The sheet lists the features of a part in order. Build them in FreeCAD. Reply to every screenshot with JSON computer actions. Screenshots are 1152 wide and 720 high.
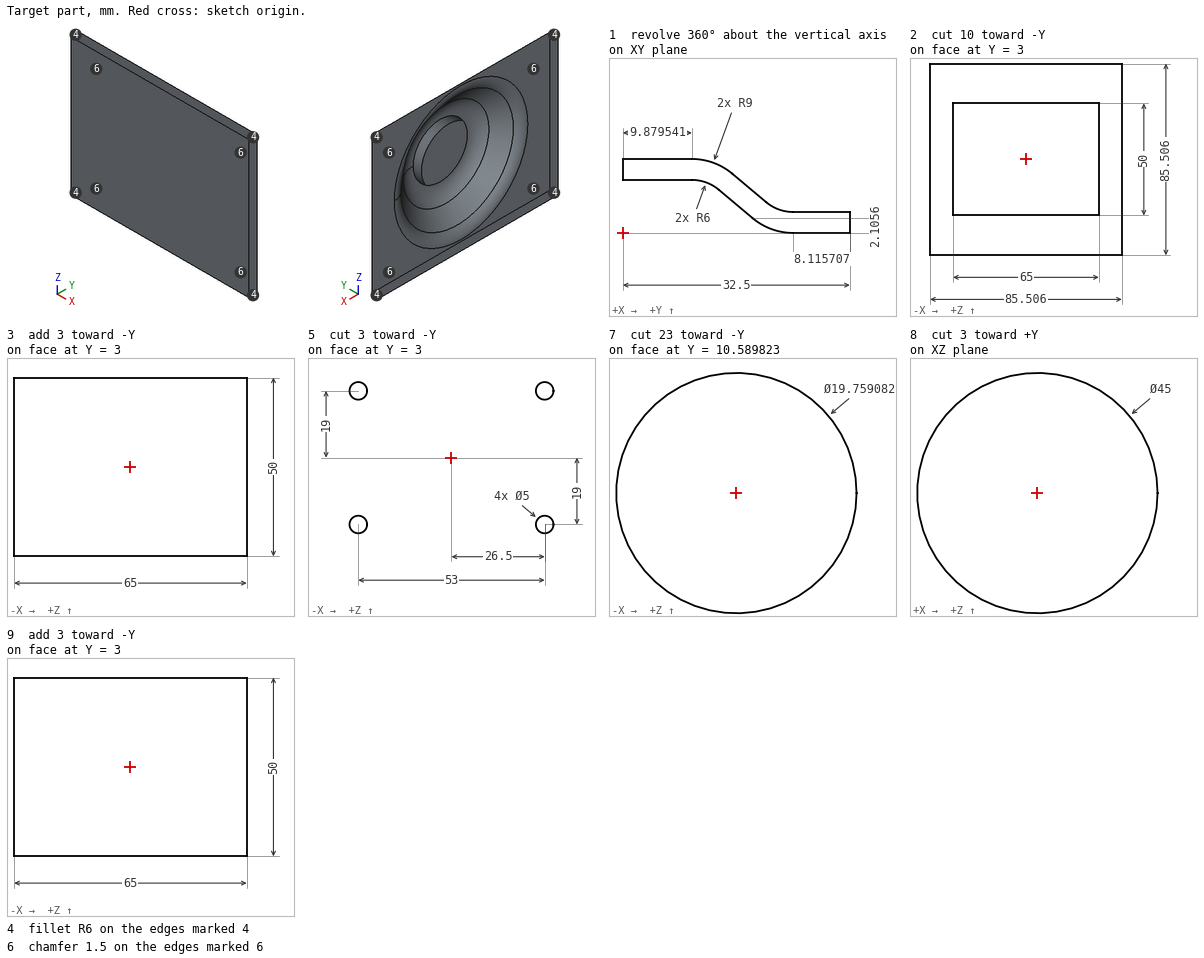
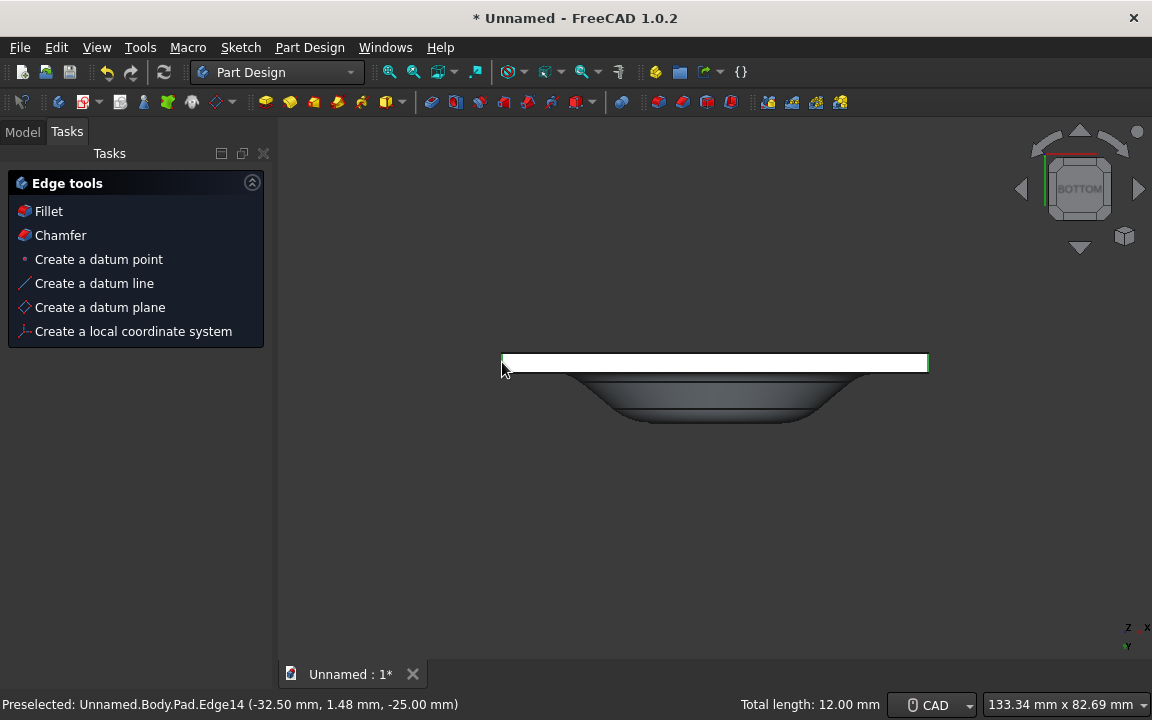
{"action": "left_click", "coordinate": [660, 102]}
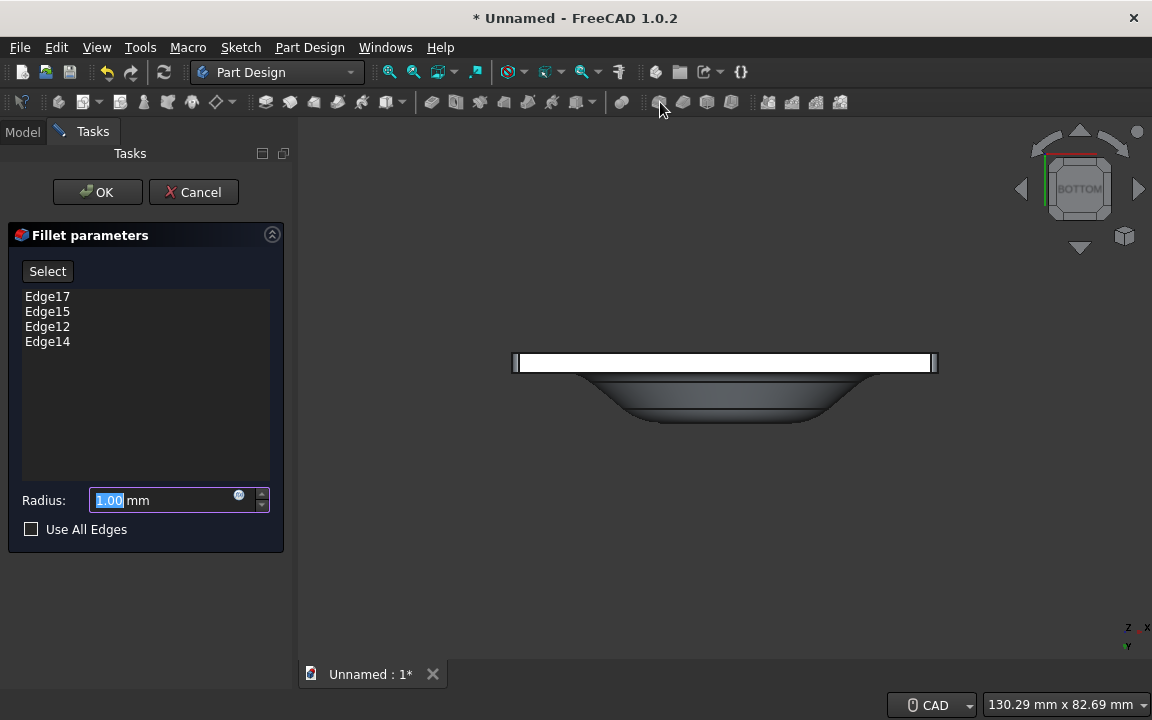
{"action": "type", "text": "6"}
{"action": "key", "text": "Tab"}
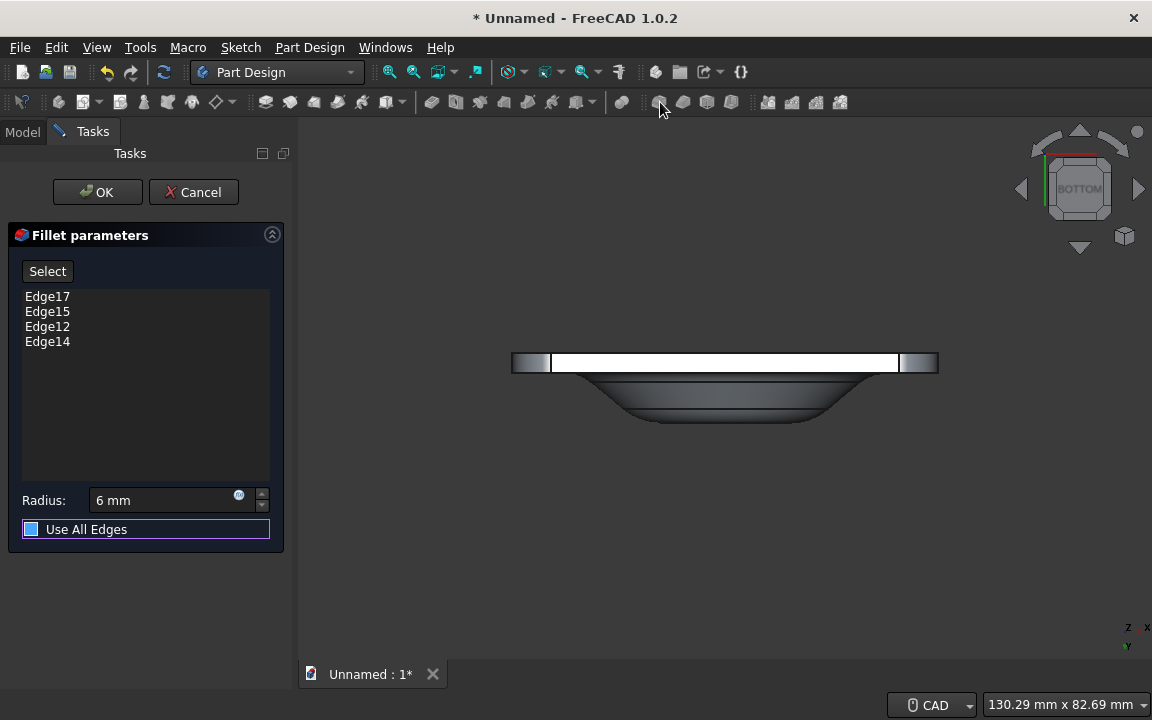
{"action": "left_click", "coordinate": [98, 192]}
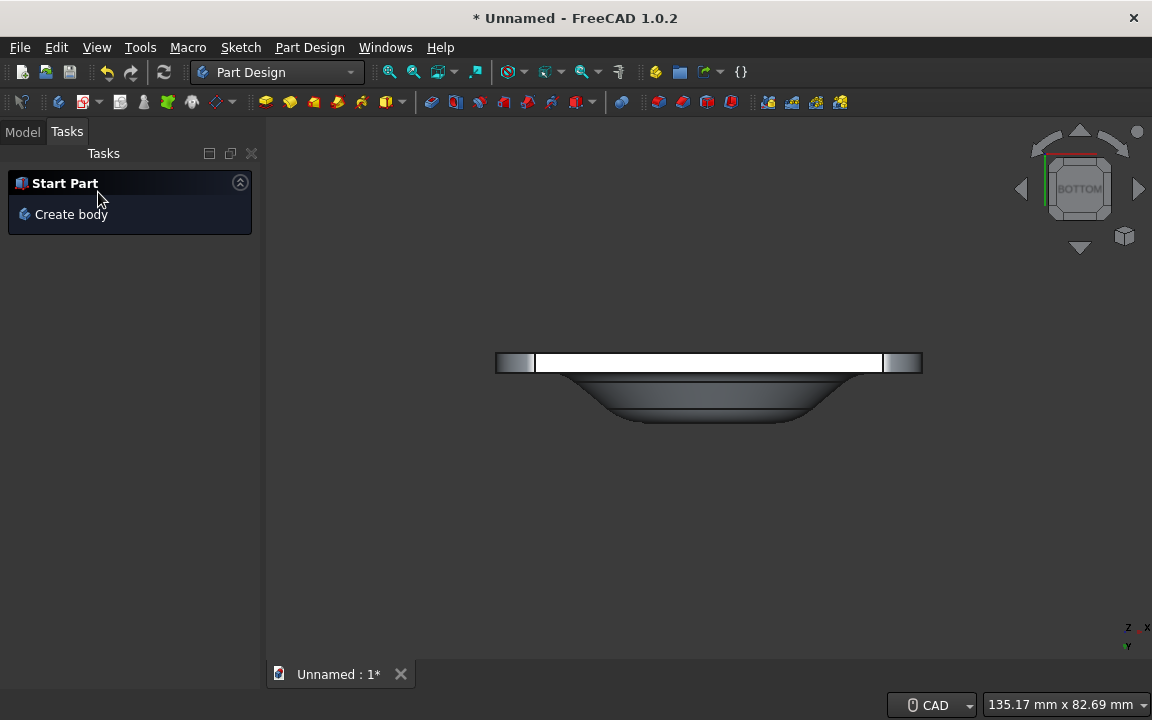
{"action": "key", "text": "4"}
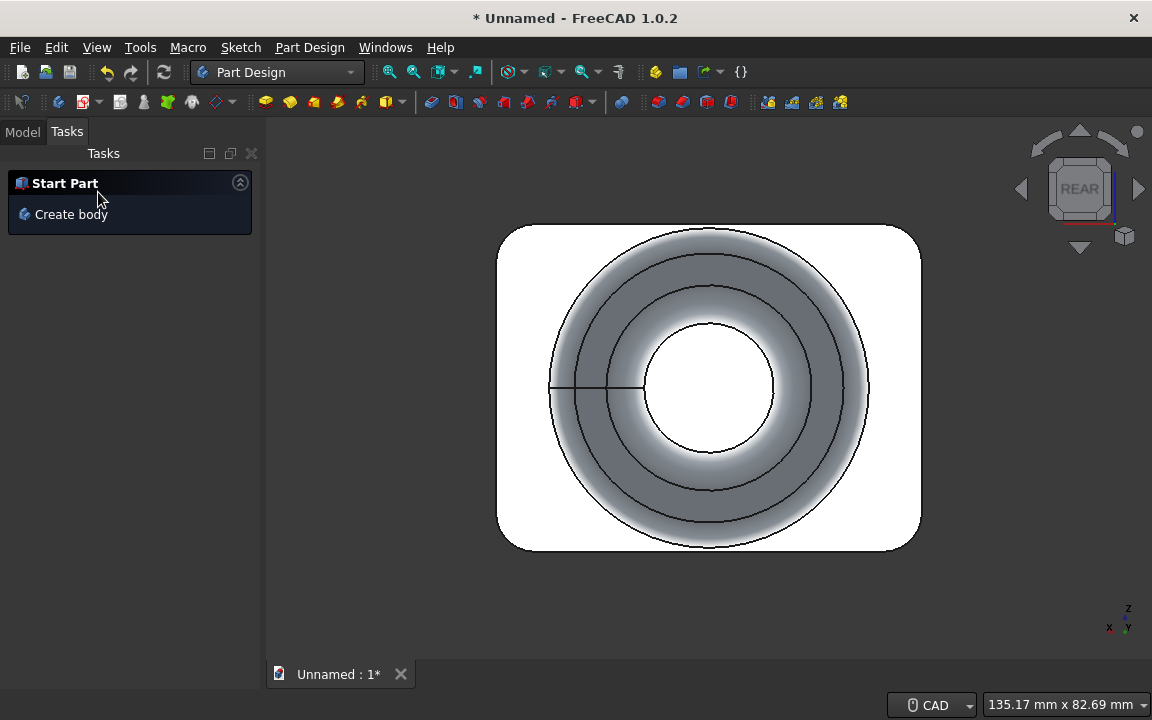
{"action": "left_click", "coordinate": [526, 293]}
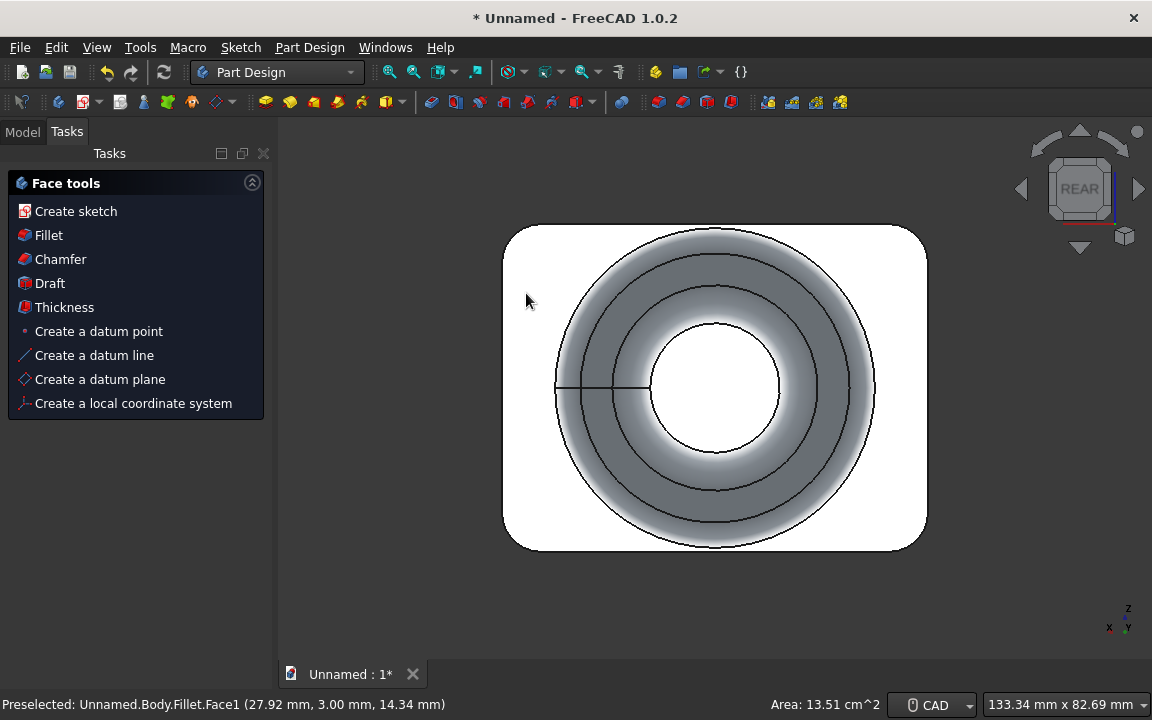
{"action": "left_click", "coordinate": [84, 102]}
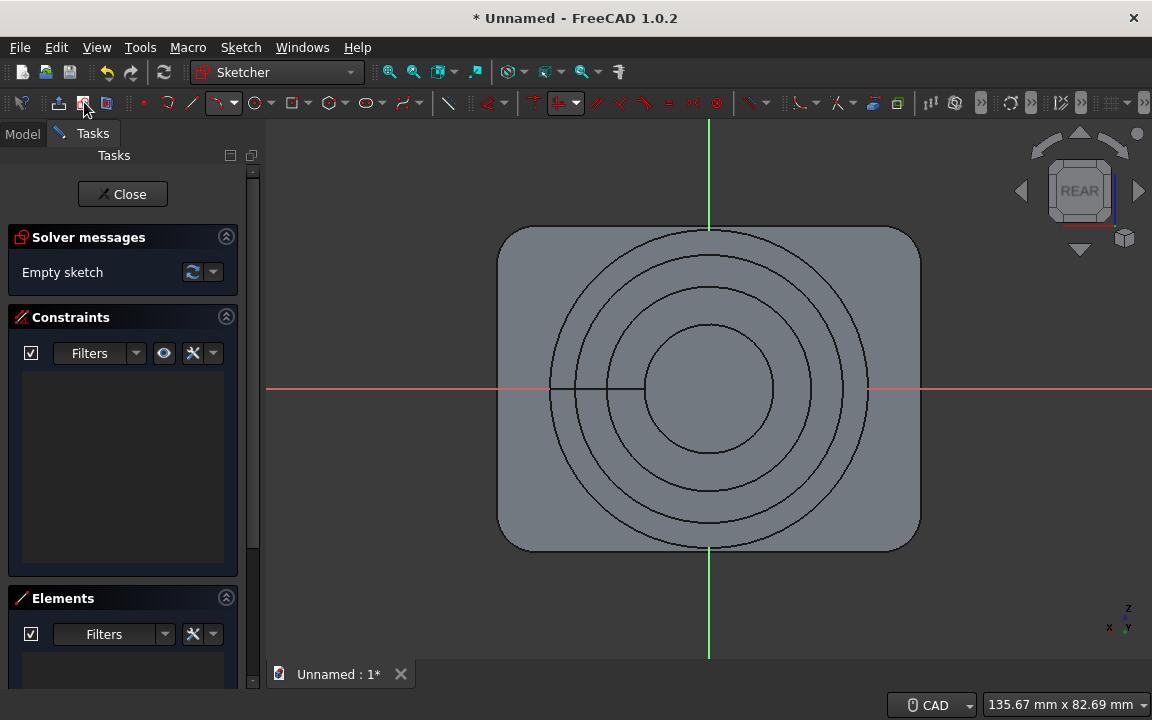
{"action": "left_click", "coordinate": [108, 104]}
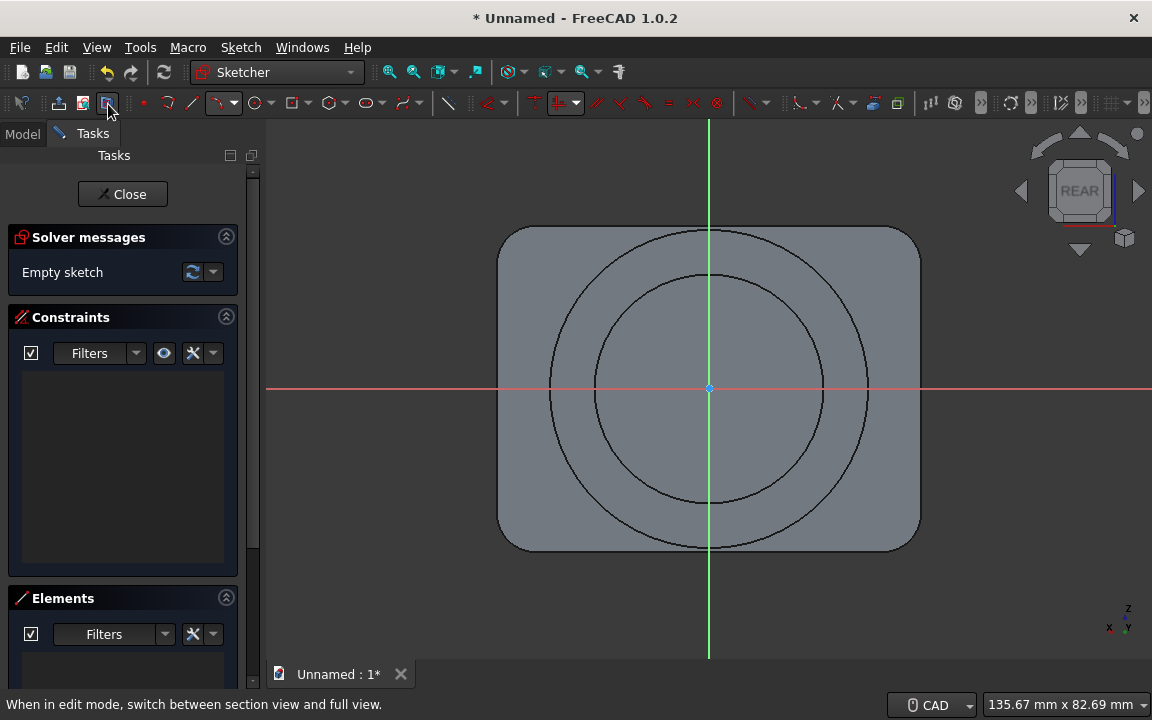
{"action": "left_click", "coordinate": [256, 104]}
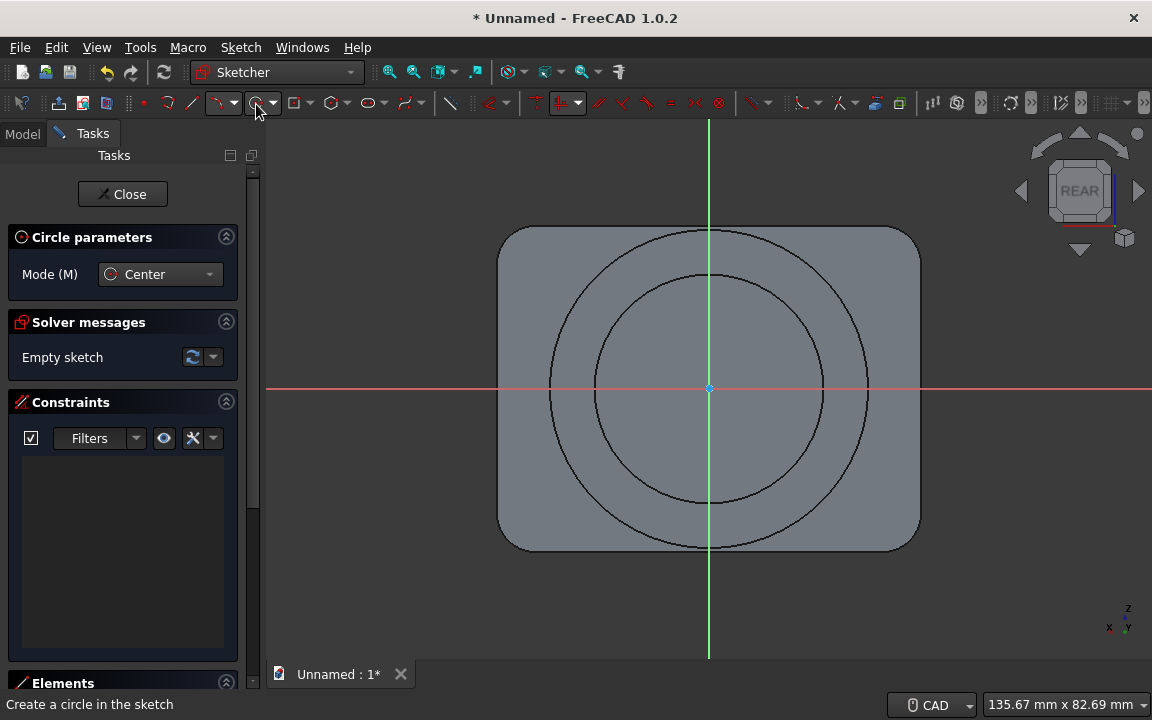
{"action": "scroll", "coordinate": [882, 513], "scroll_direction": "up", "scroll_amount": 2}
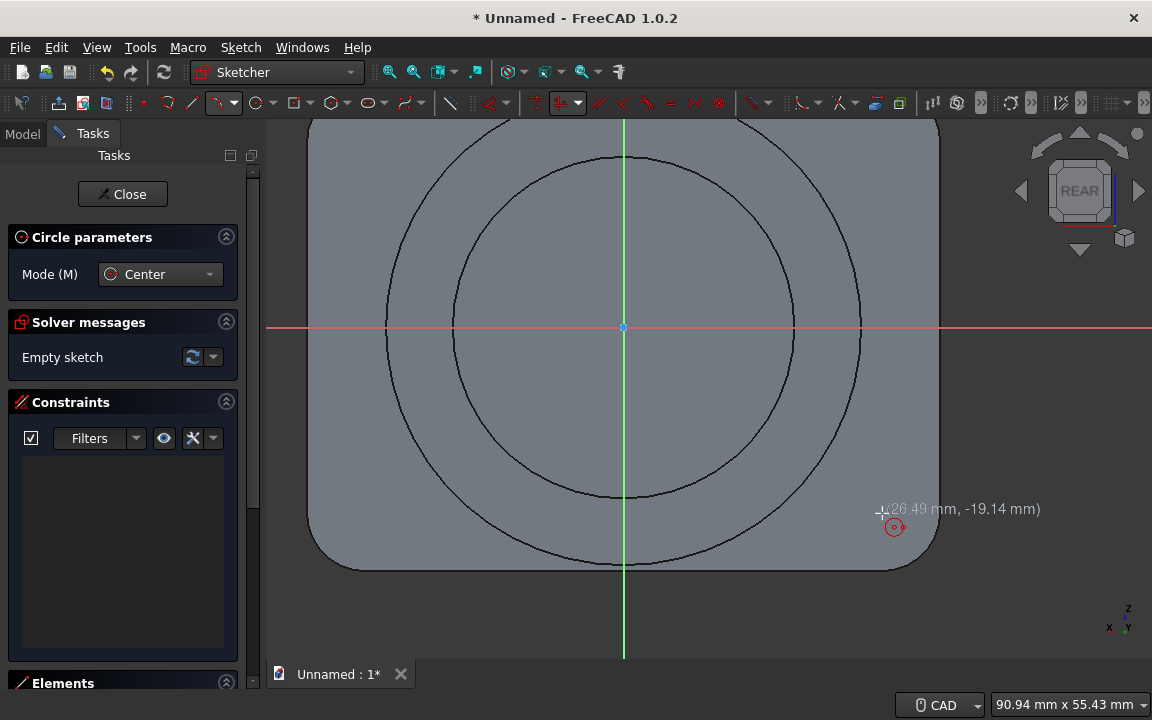
{"action": "left_click", "coordinate": [882, 513]}
{"action": "left_click", "coordinate": [899, 496]}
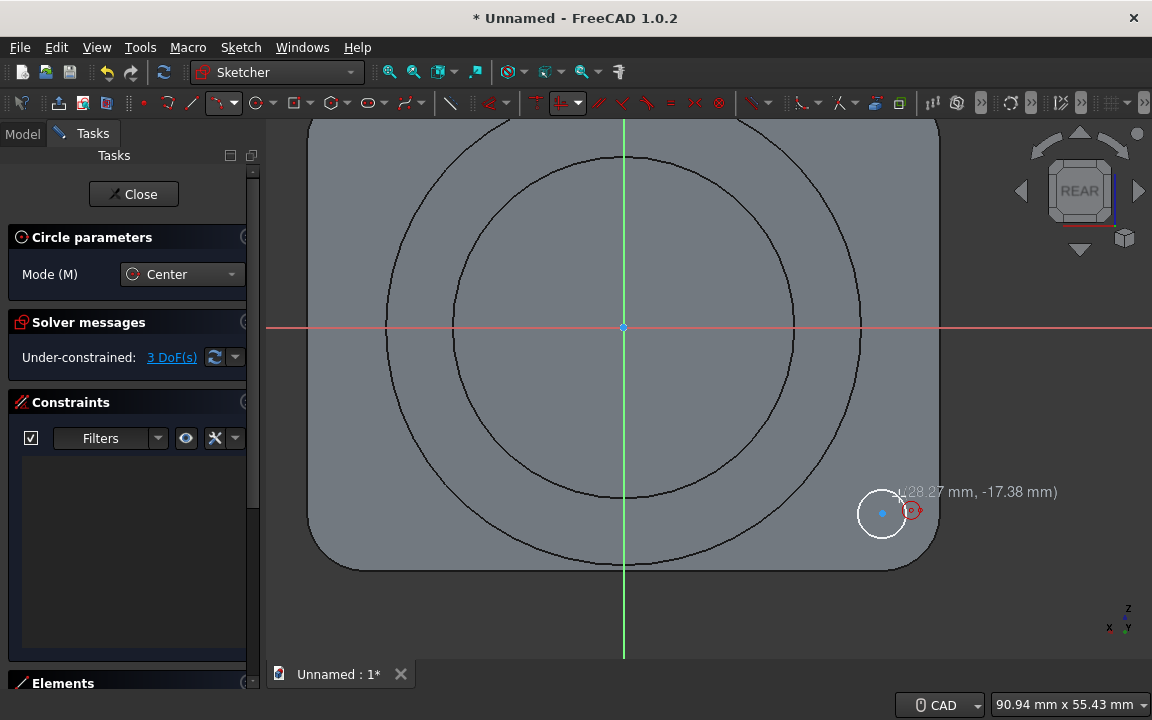
{"action": "left_click", "coordinate": [365, 513]}
{"action": "left_click", "coordinate": [383, 496]}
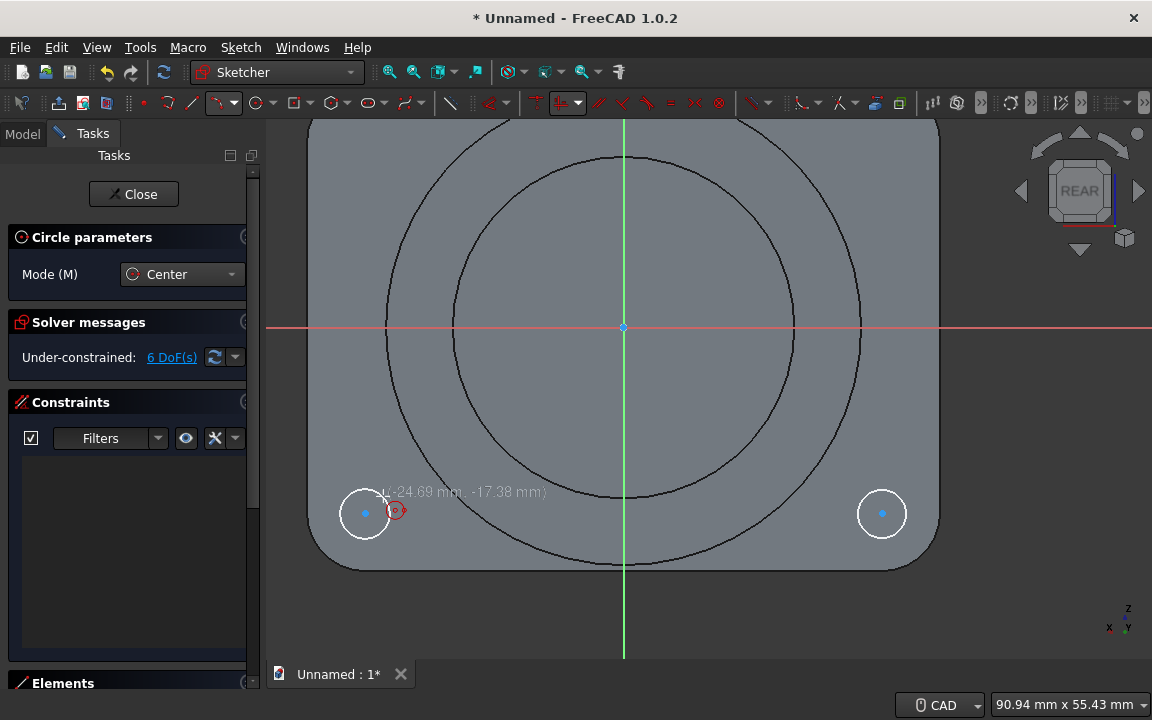
{"action": "scroll", "coordinate": [717, 631], "scroll_direction": "down", "scroll_amount": 1}